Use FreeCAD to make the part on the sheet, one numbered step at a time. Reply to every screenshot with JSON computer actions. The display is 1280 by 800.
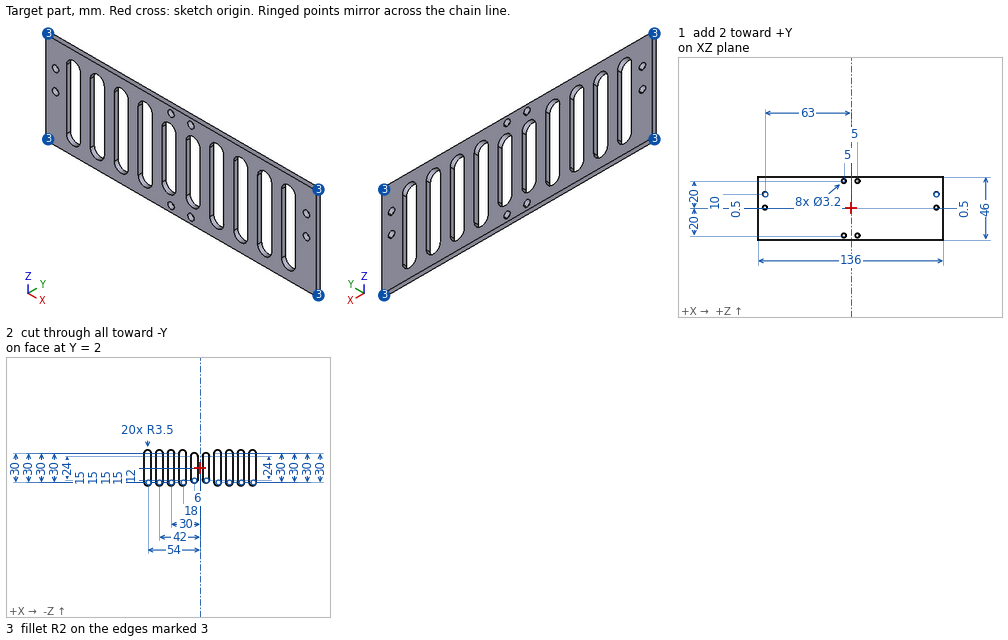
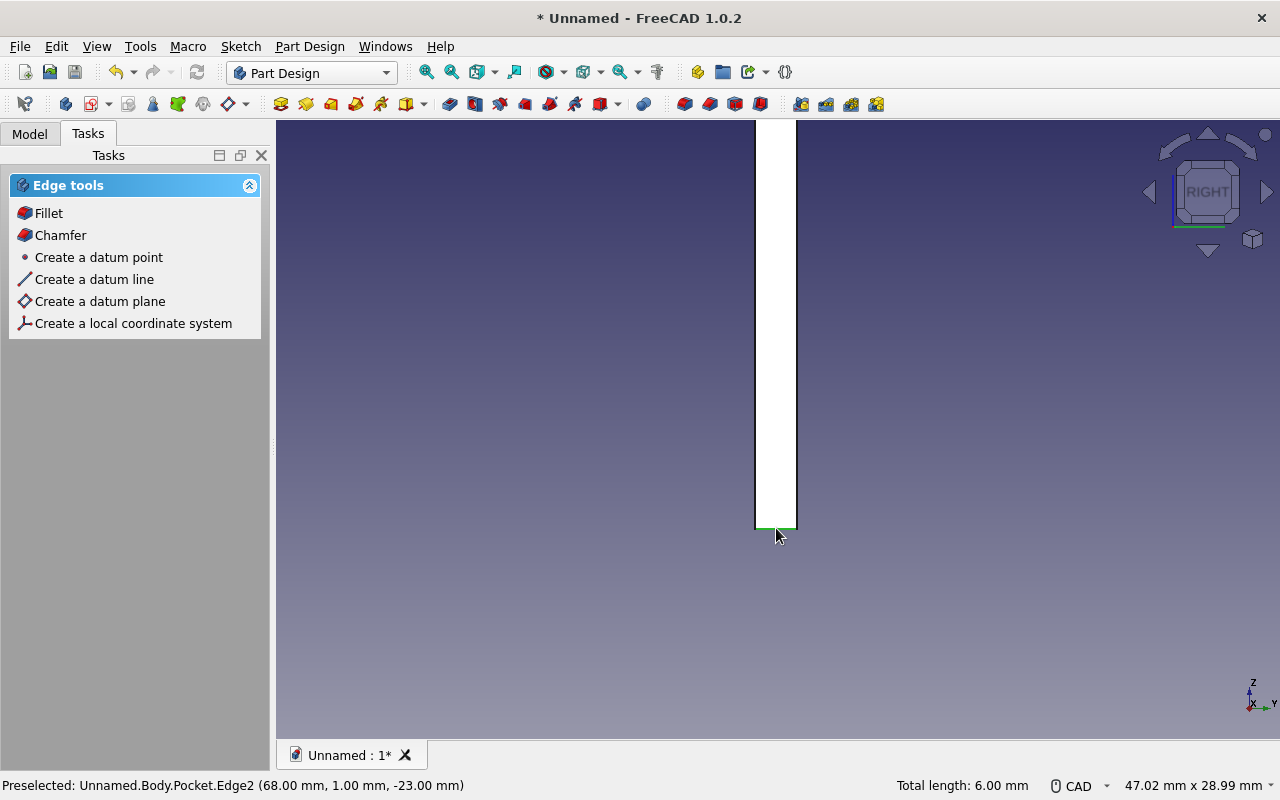
{"action": "left_click", "coordinate": [427, 72]}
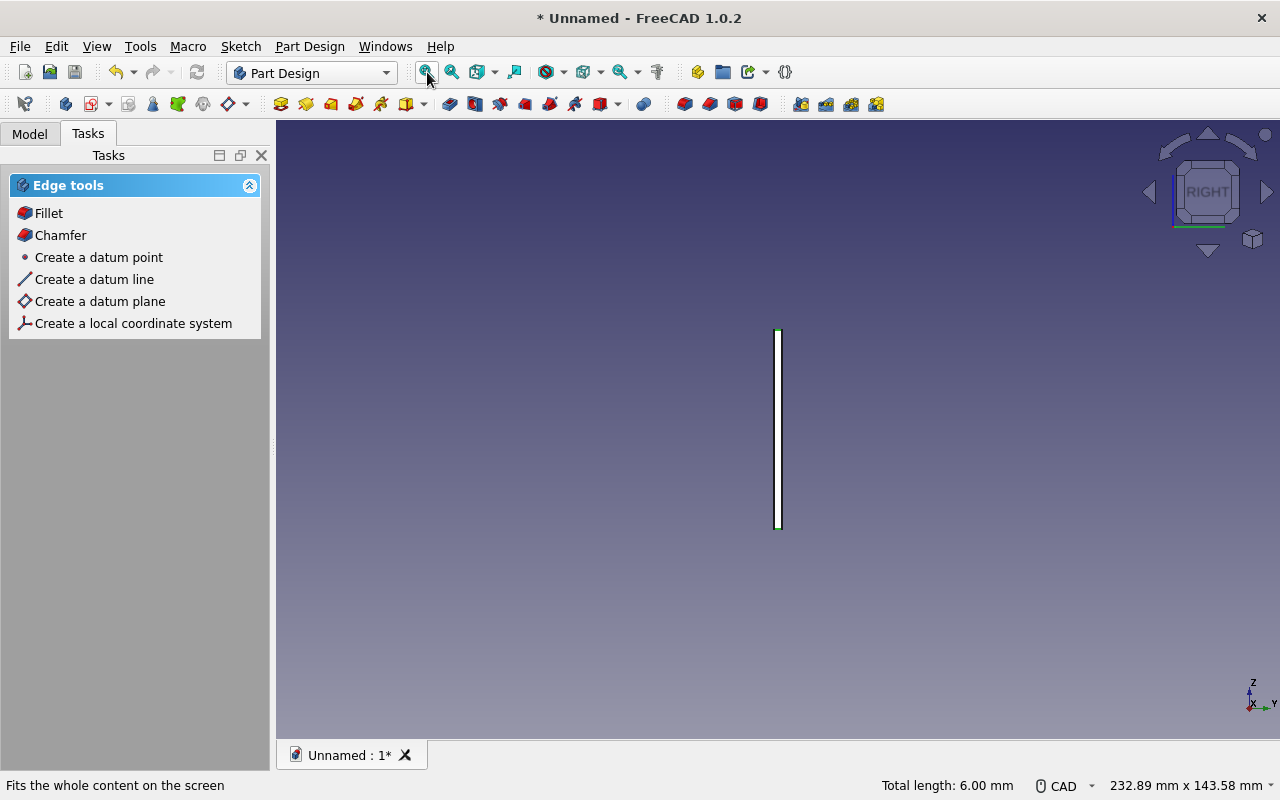
{"action": "key", "text": "5"}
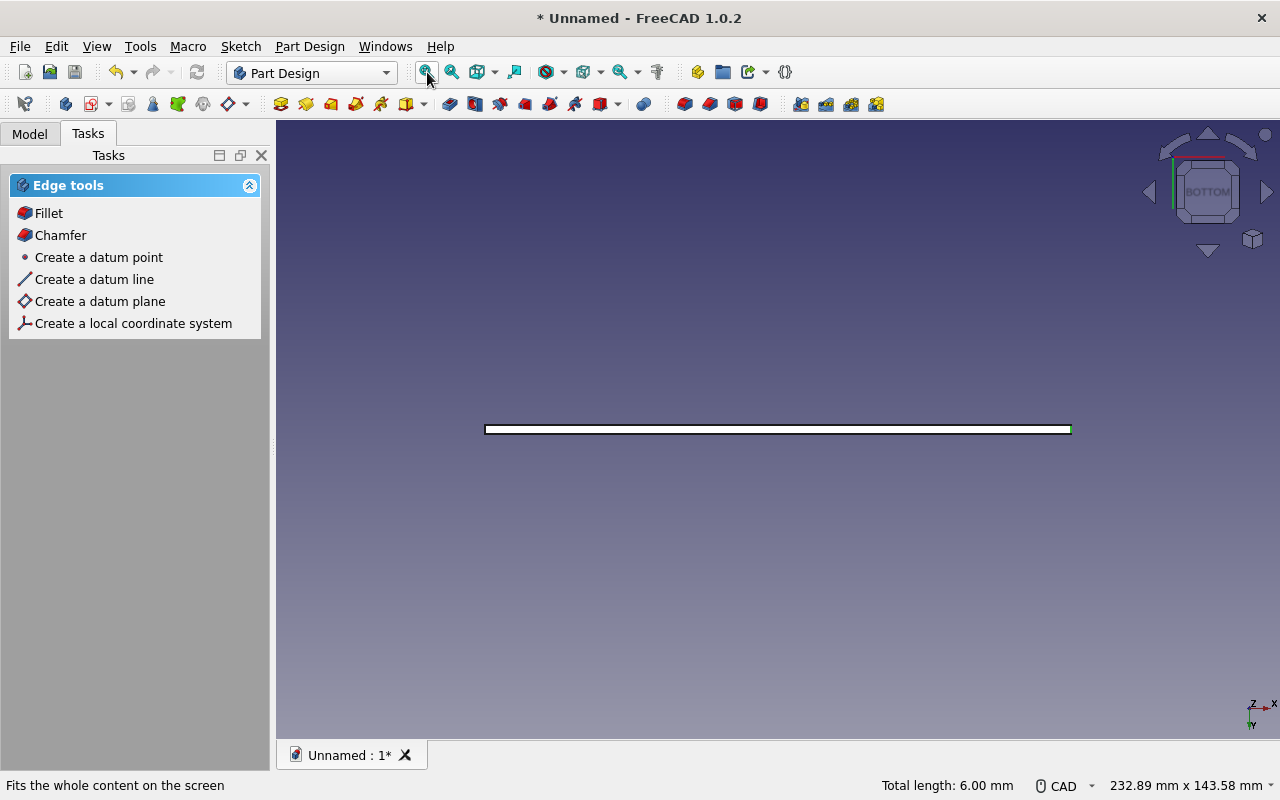
{"action": "scroll", "coordinate": [485, 428], "scroll_direction": "up", "scroll_amount": 8}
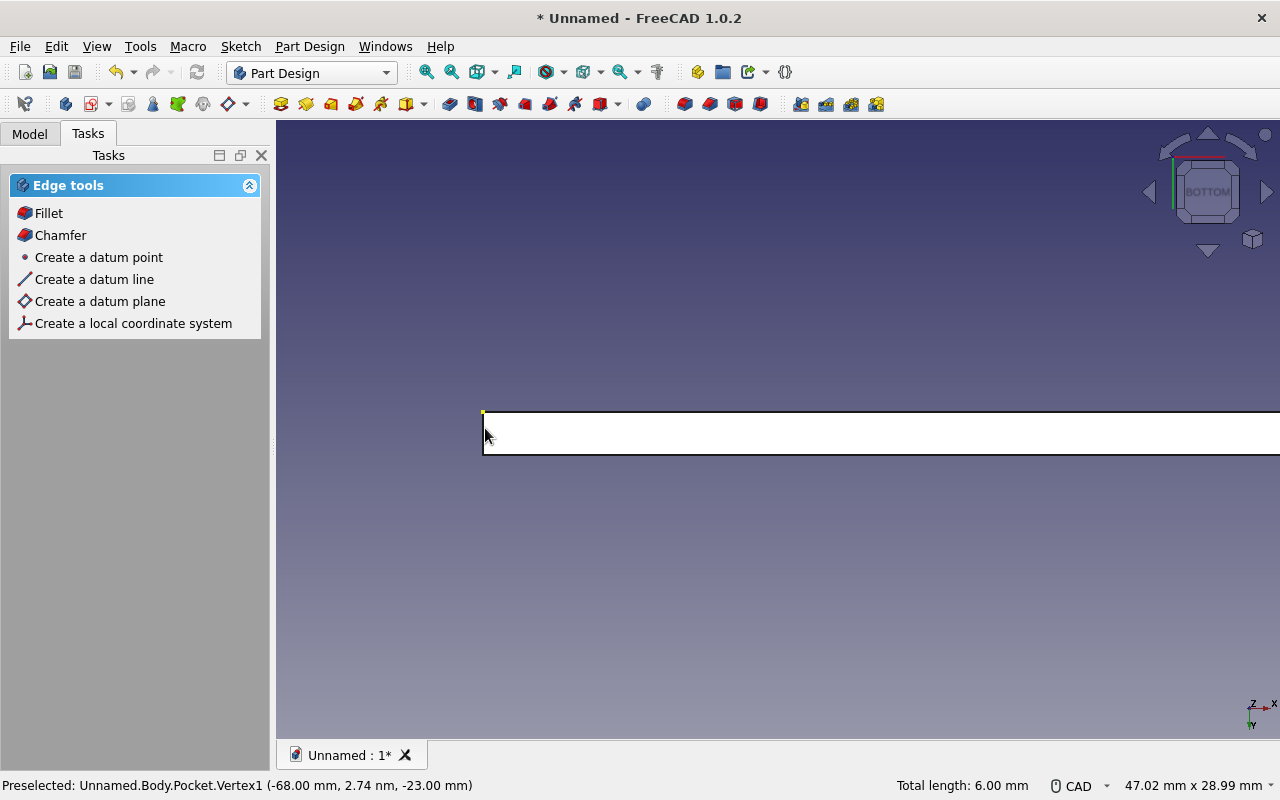
{"action": "left_click", "coordinate": [483, 432], "text": "ctrl"}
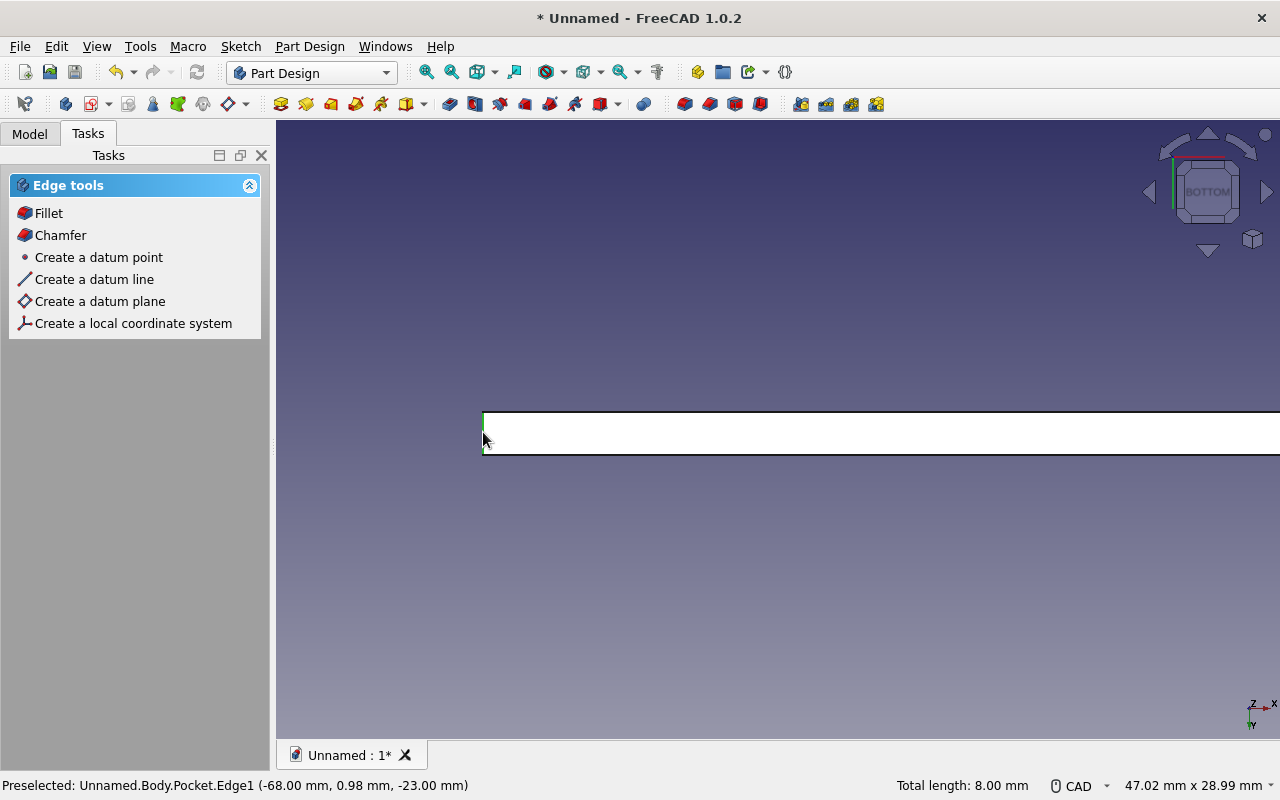
{"action": "left_click", "coordinate": [685, 104]}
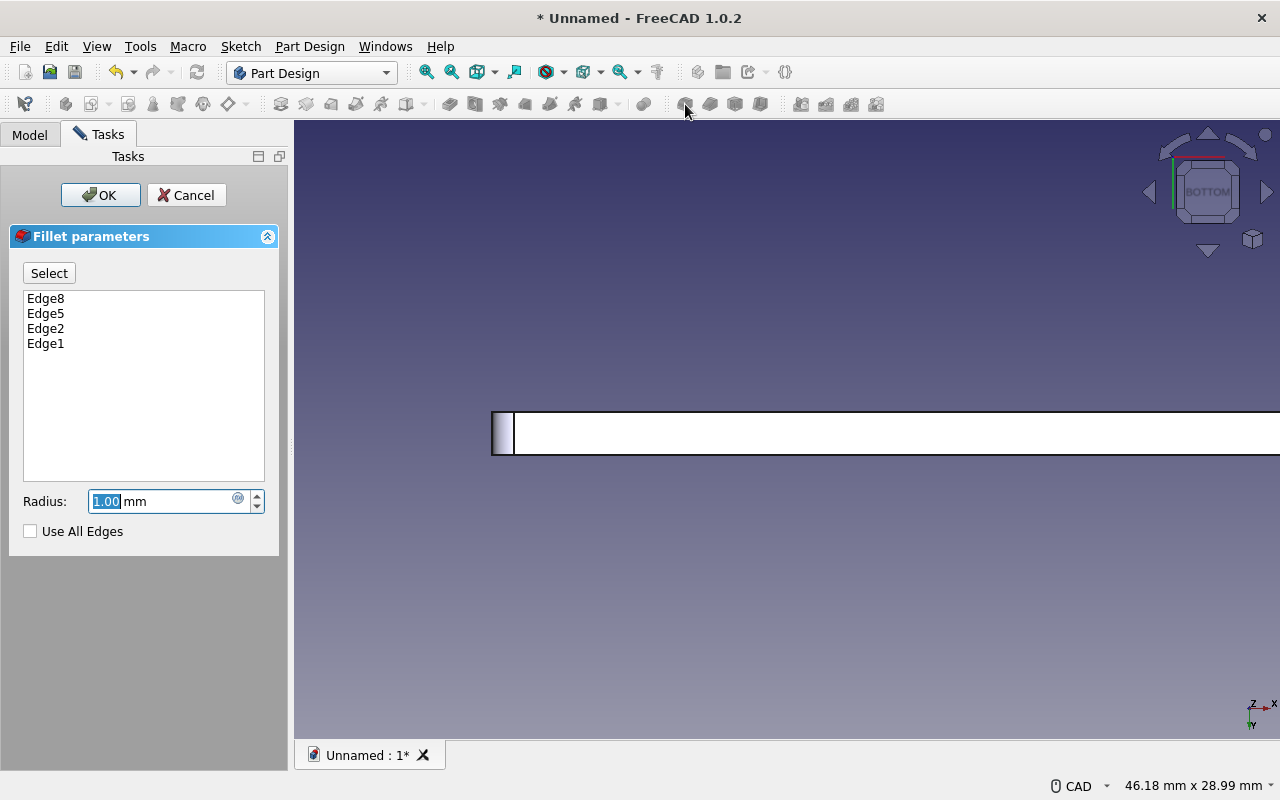
{"action": "type", "text": "2"}
{"action": "key", "text": "Tab"}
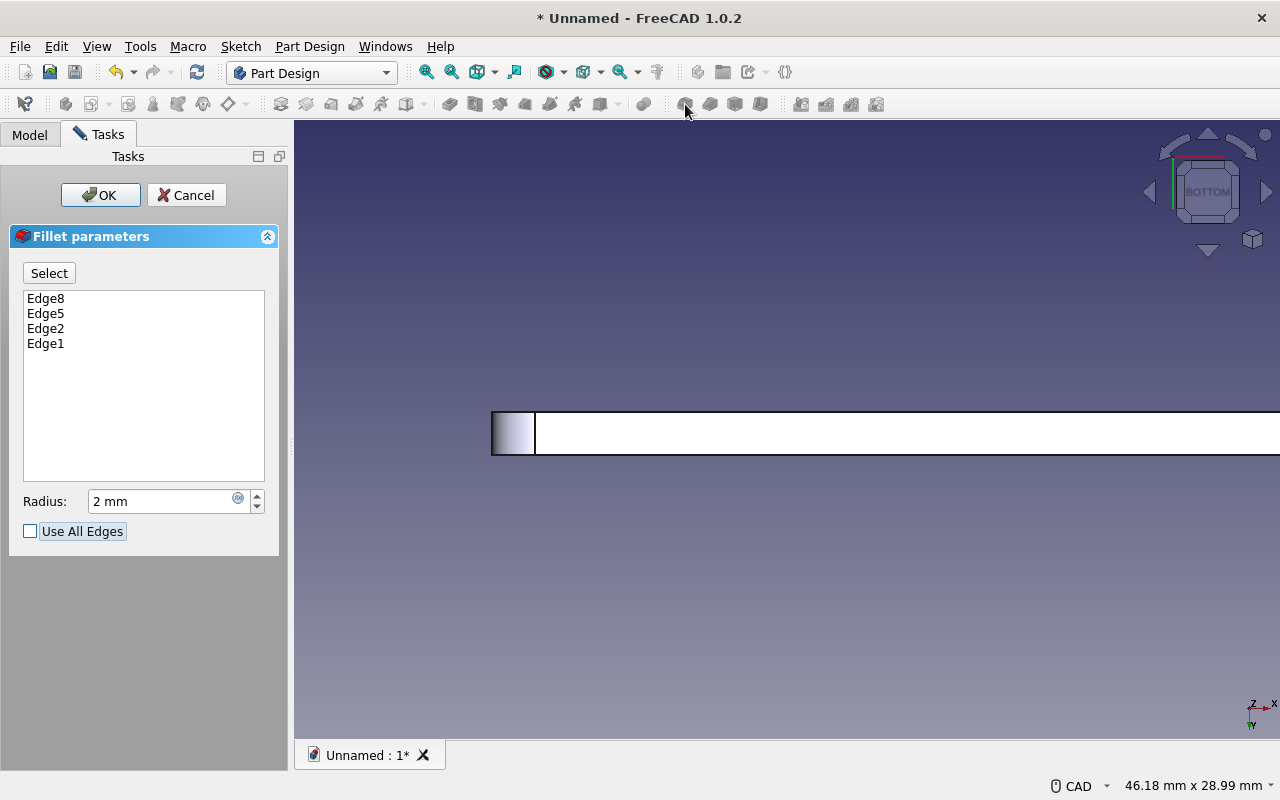
{"action": "left_click", "coordinate": [101, 195]}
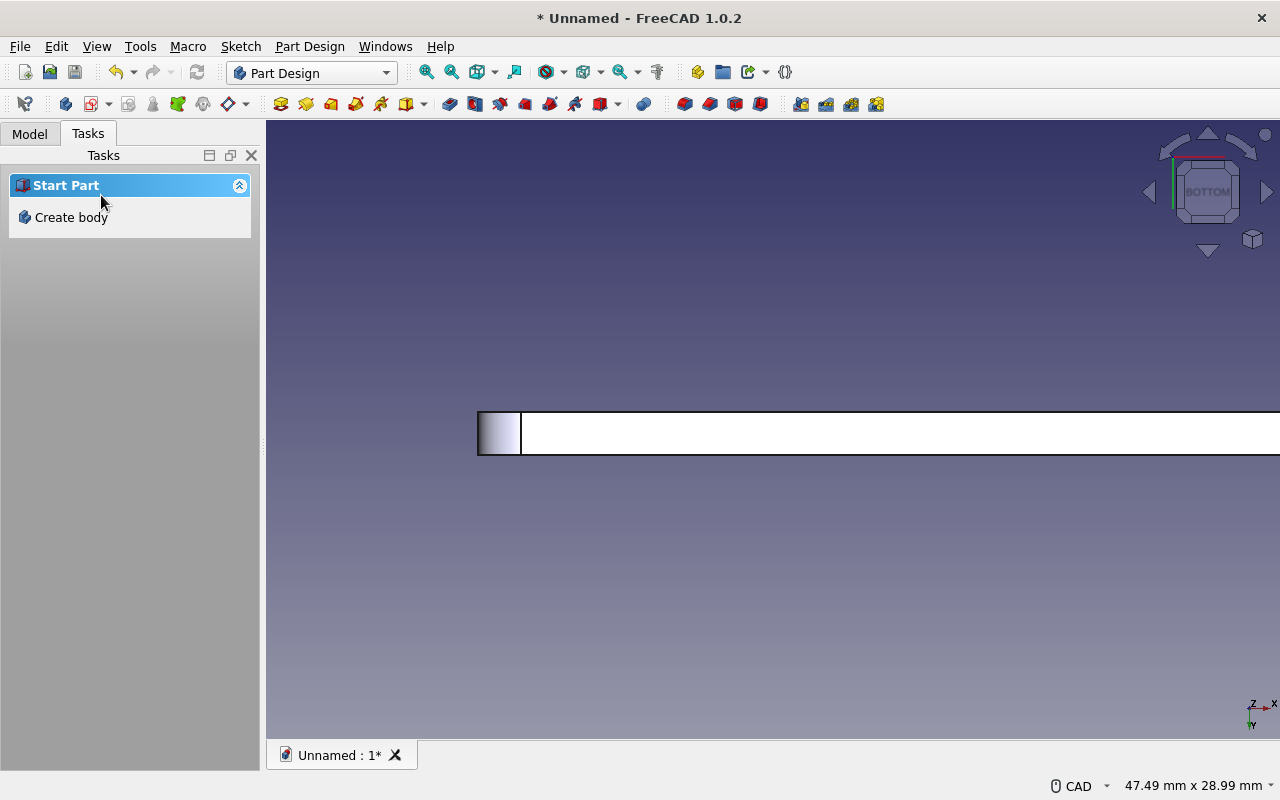
{"action": "key", "text": "0"}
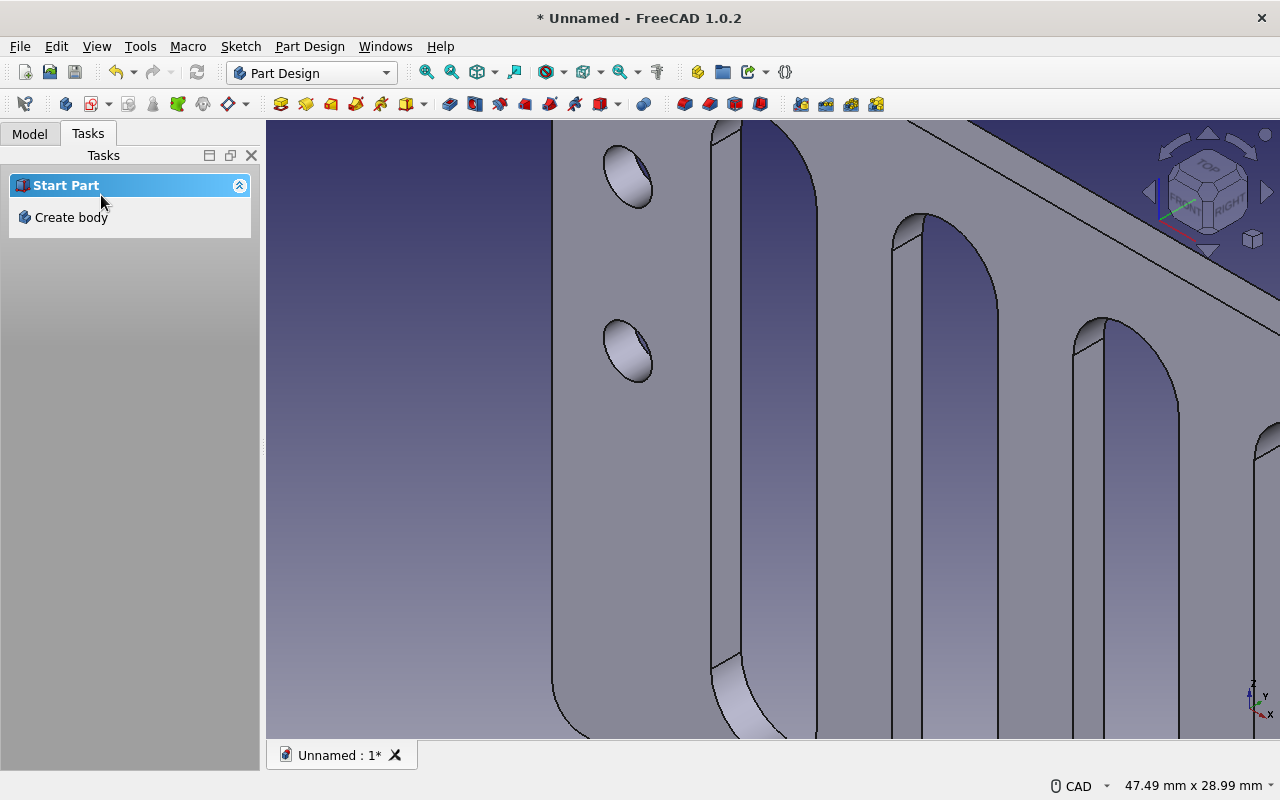
{"action": "left_click", "coordinate": [427, 72]}